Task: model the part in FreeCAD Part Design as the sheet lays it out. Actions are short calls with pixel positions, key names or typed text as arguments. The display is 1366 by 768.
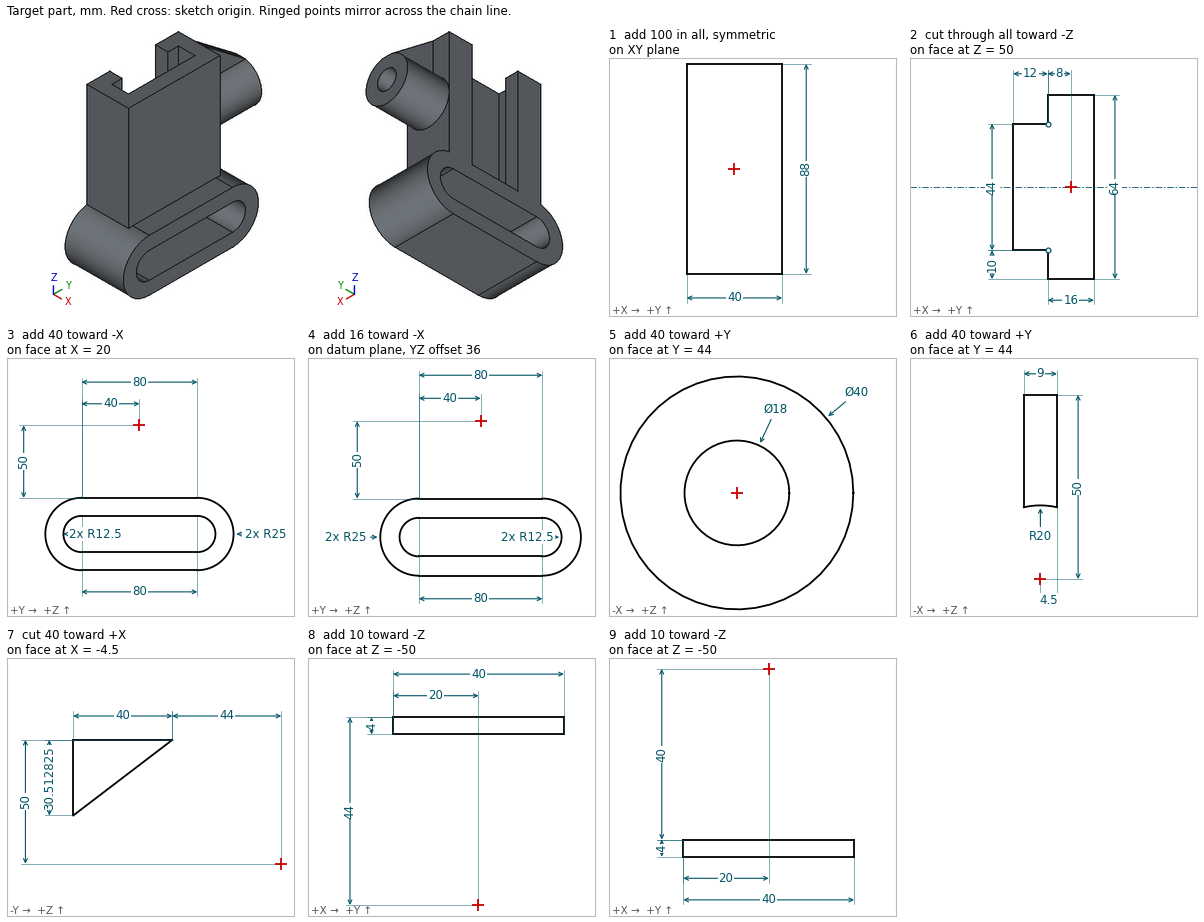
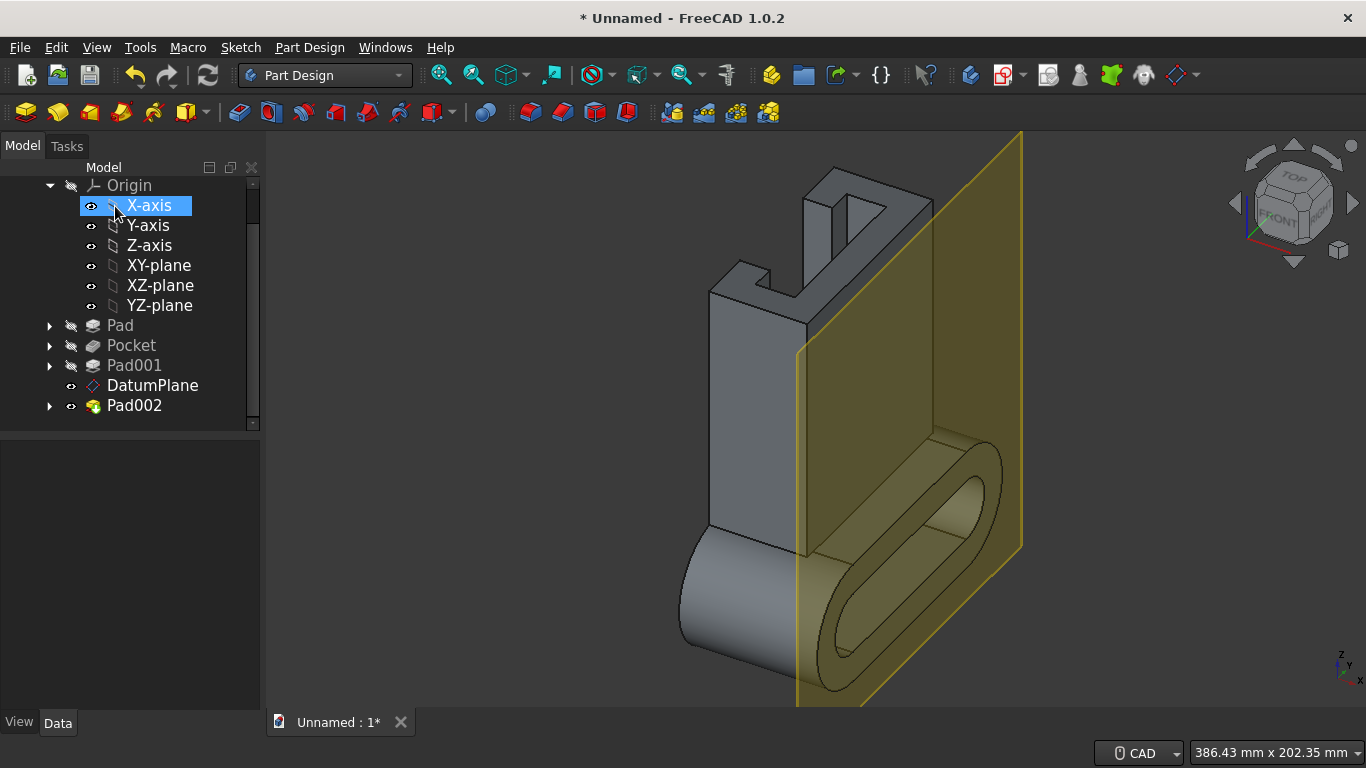
click(116, 386)
key(space)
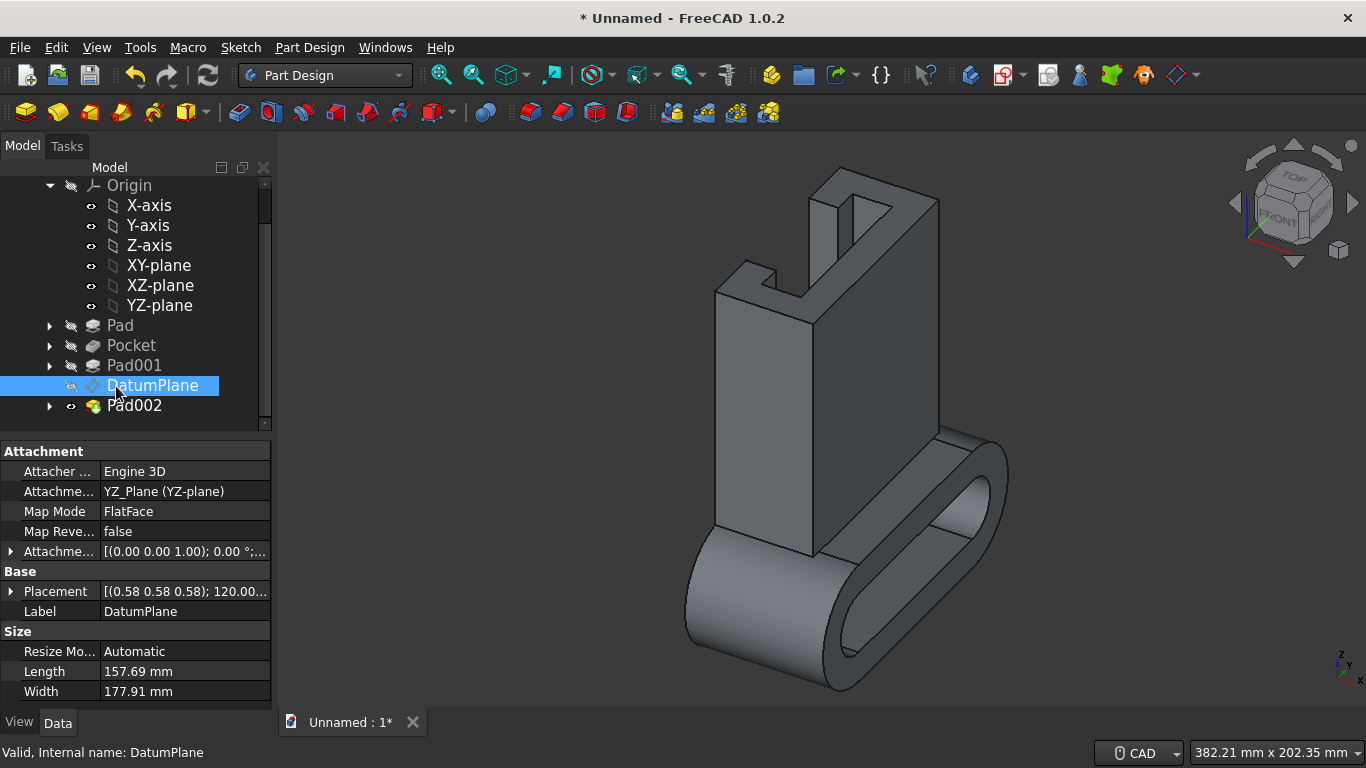
key(v)
key(f)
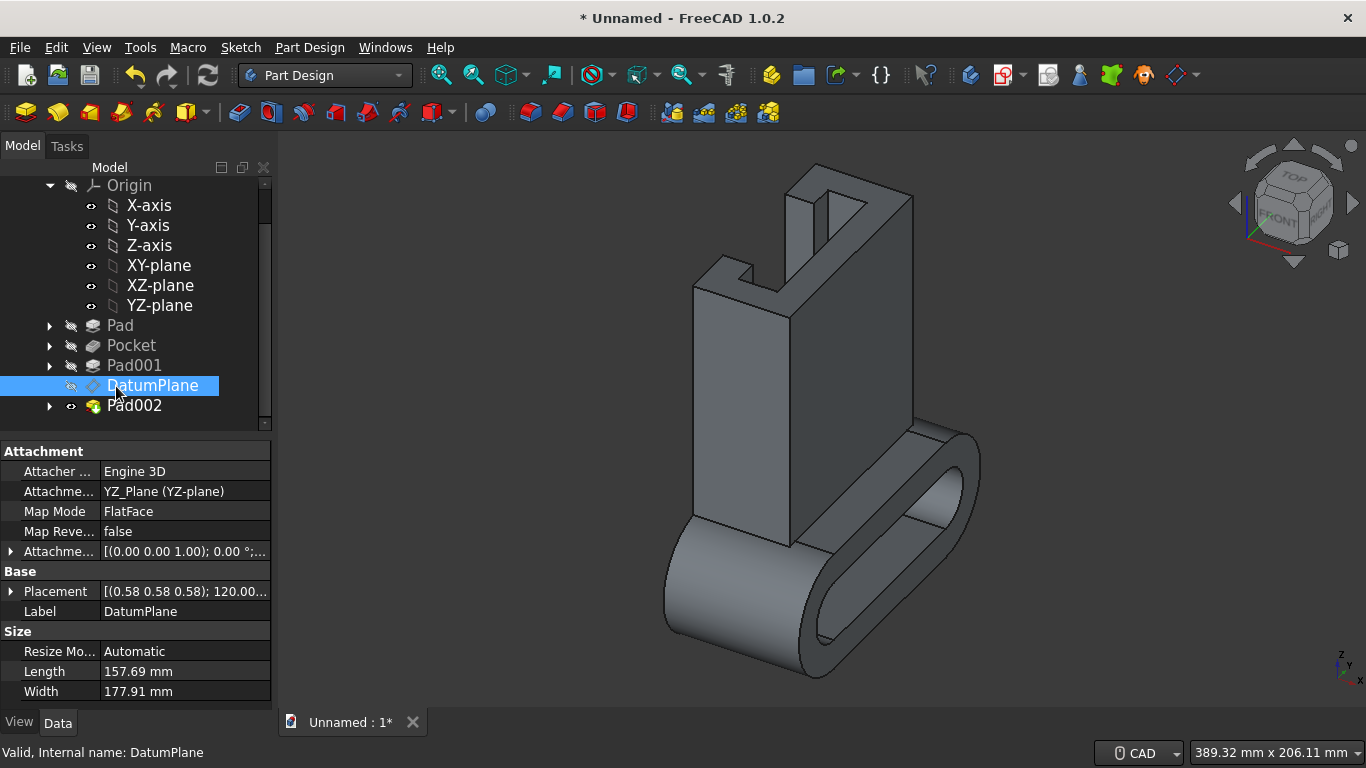
key(4)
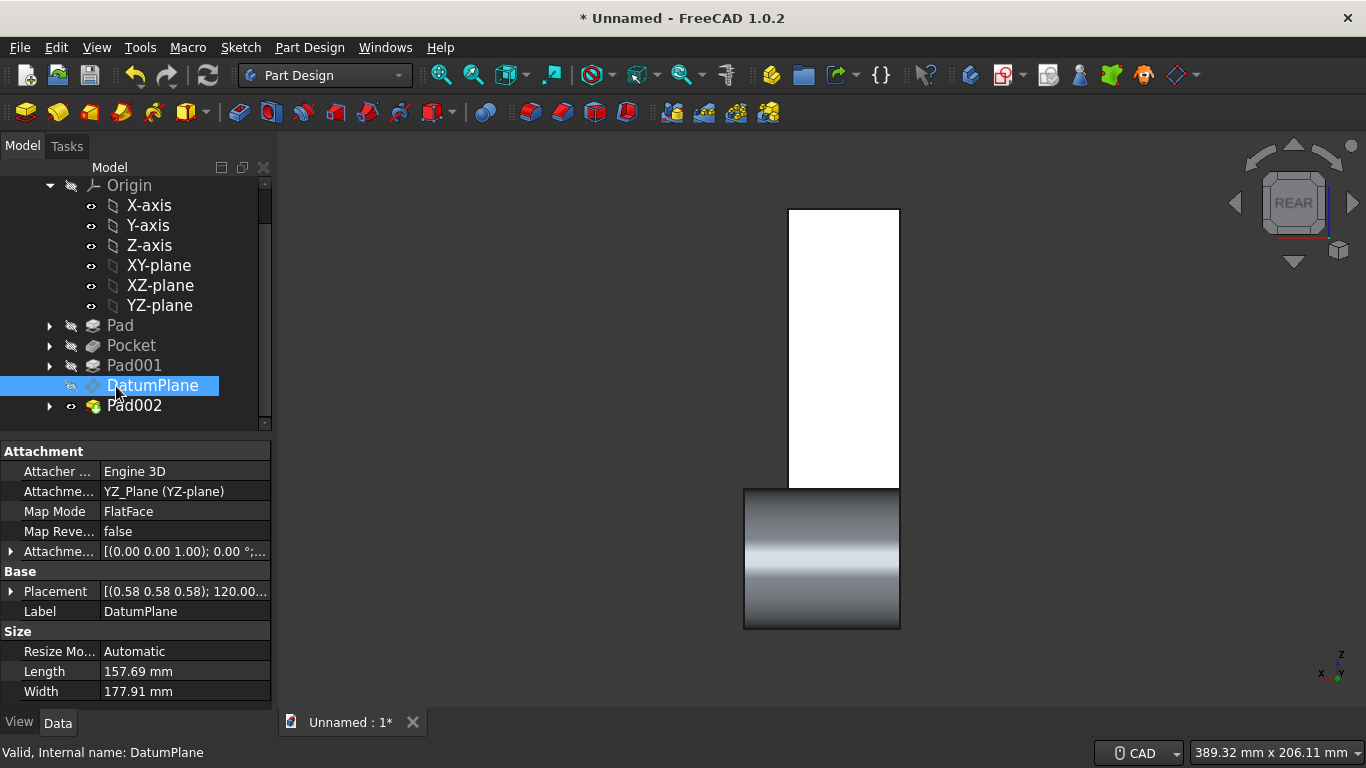
click(844, 268)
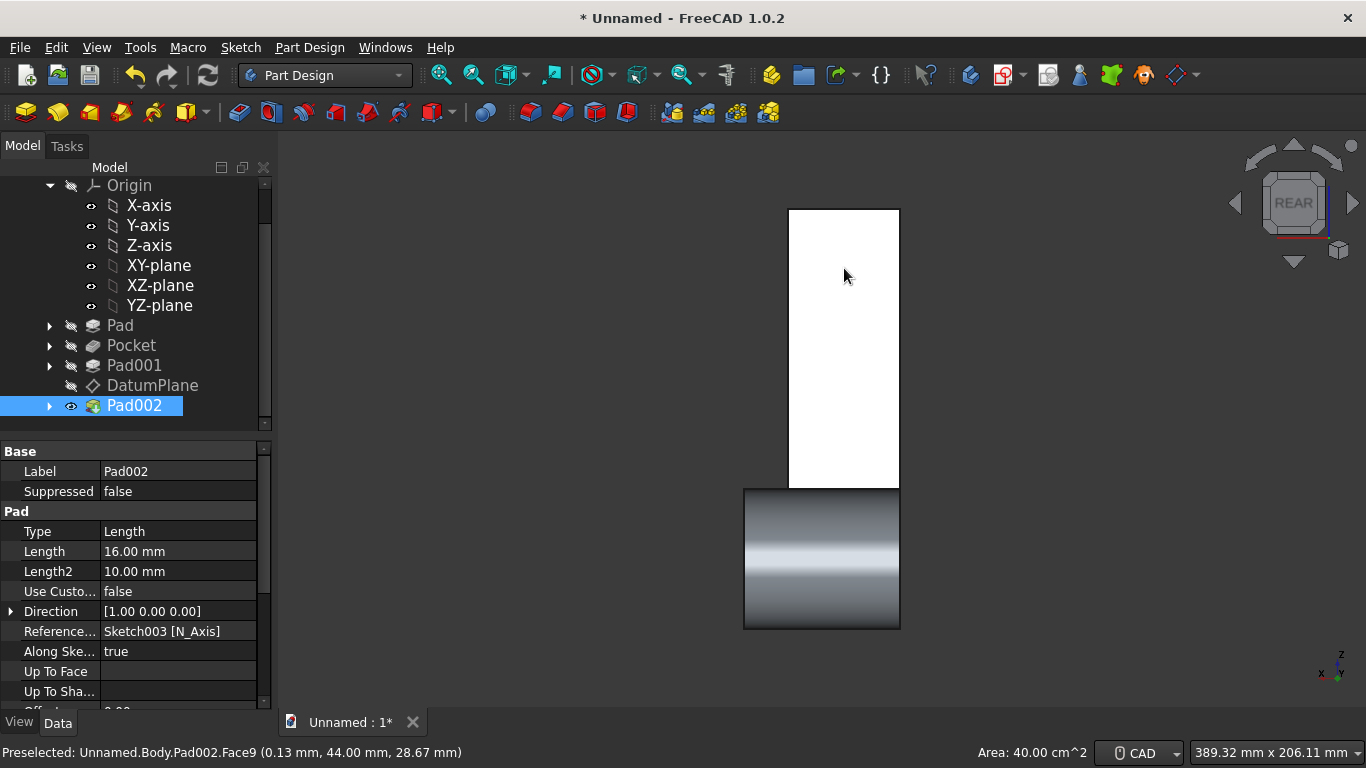
click(1004, 76)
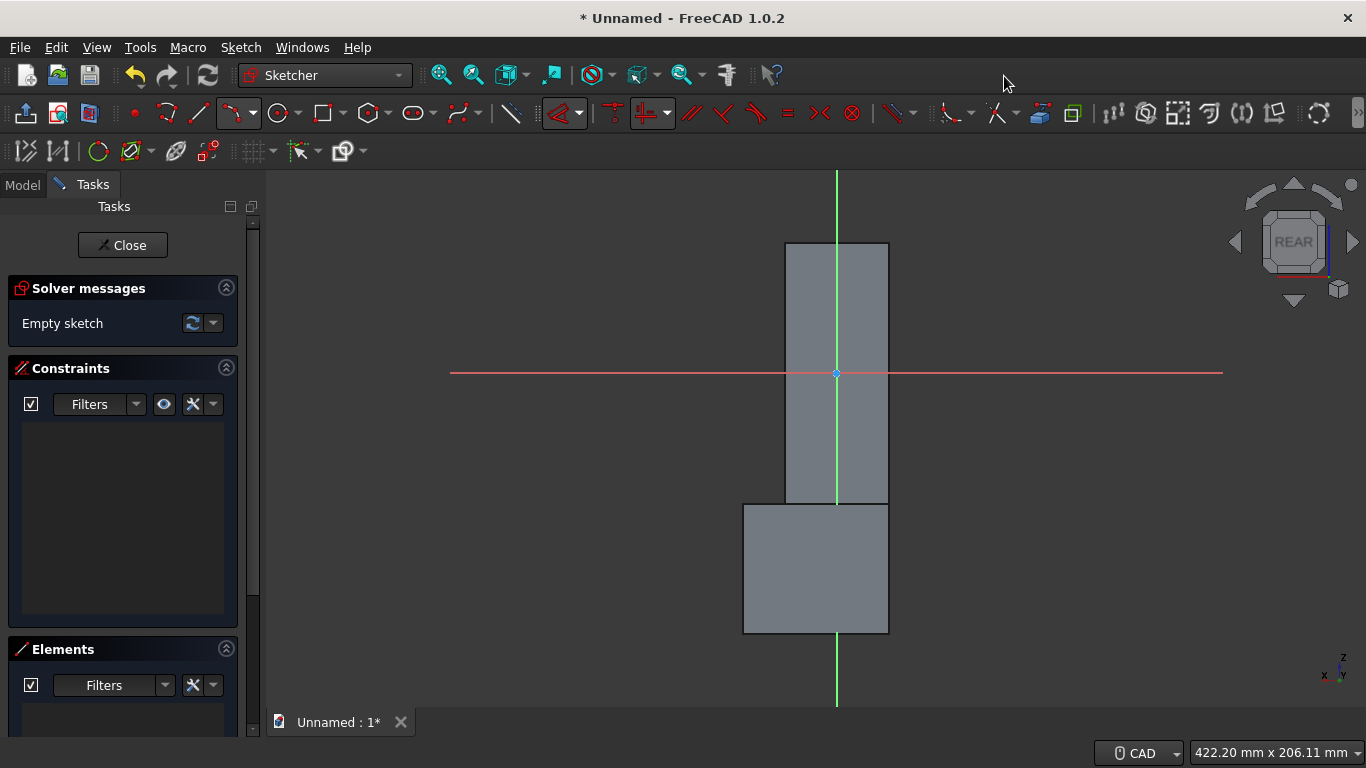
click(90, 114)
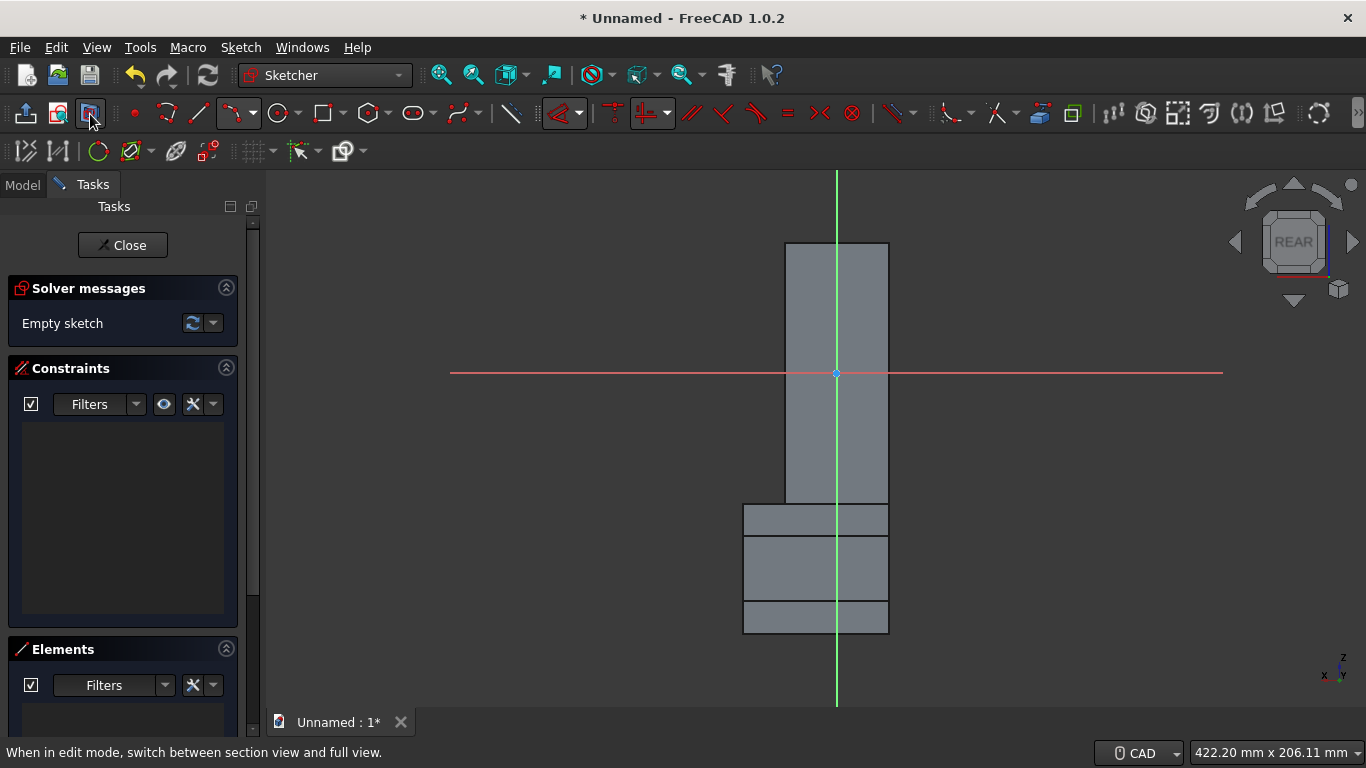
scroll(875, 345, up, 6)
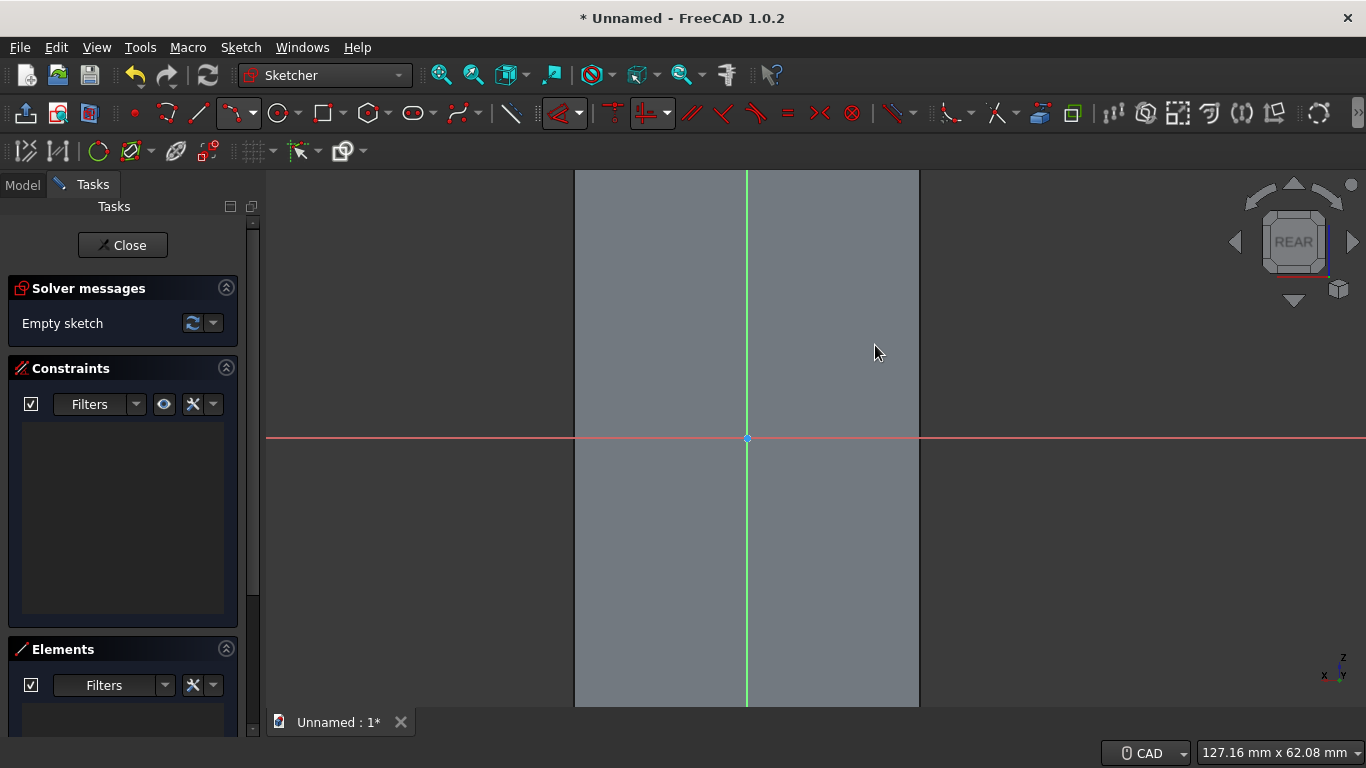
click(278, 114)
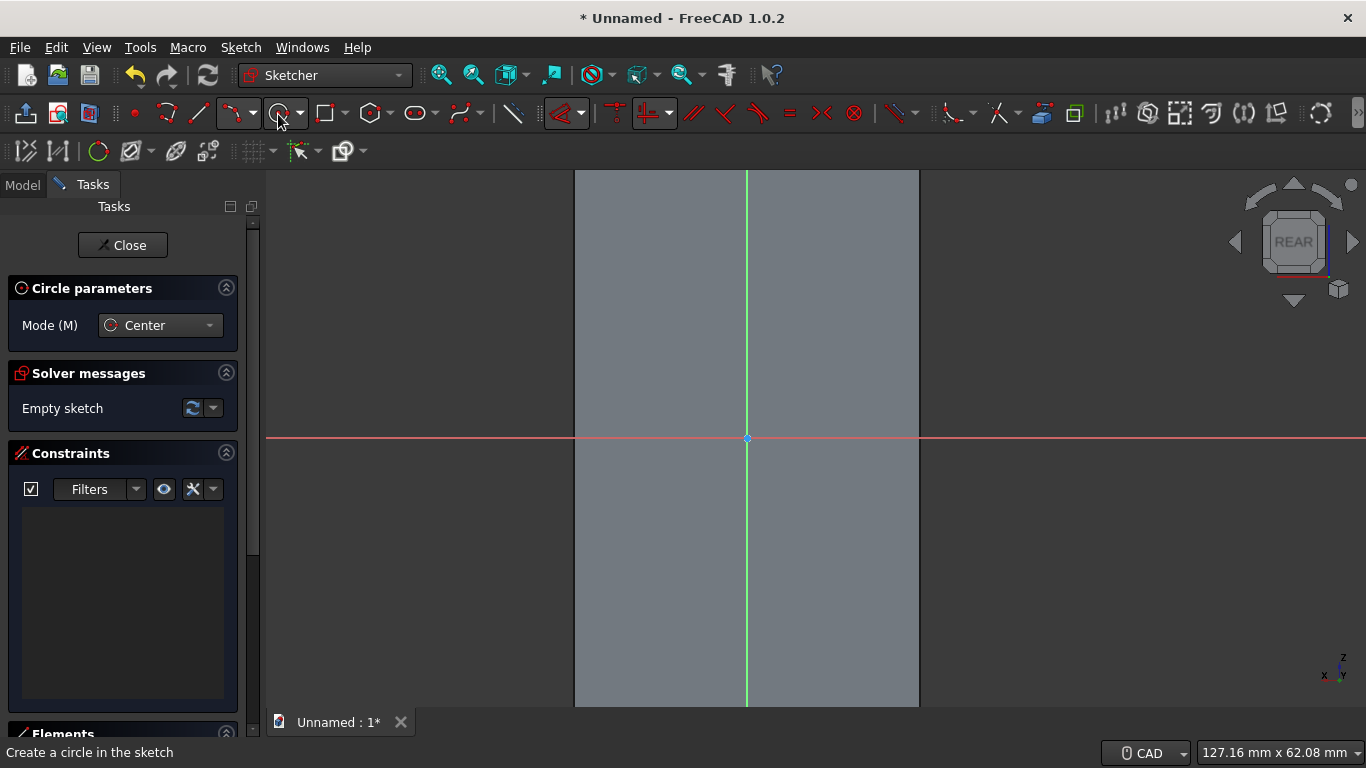
click(747, 438)
click(869, 316)